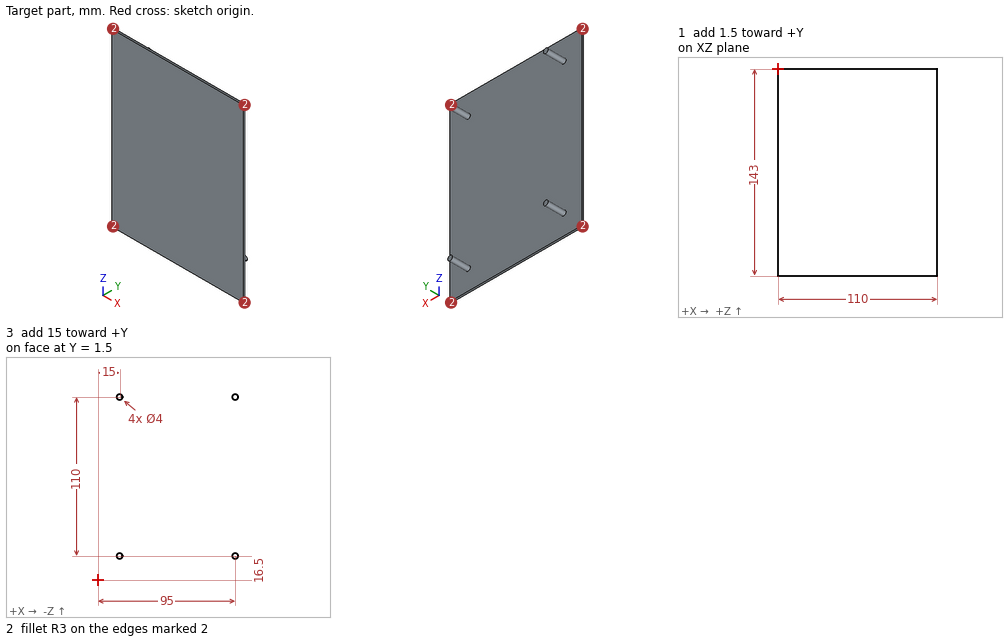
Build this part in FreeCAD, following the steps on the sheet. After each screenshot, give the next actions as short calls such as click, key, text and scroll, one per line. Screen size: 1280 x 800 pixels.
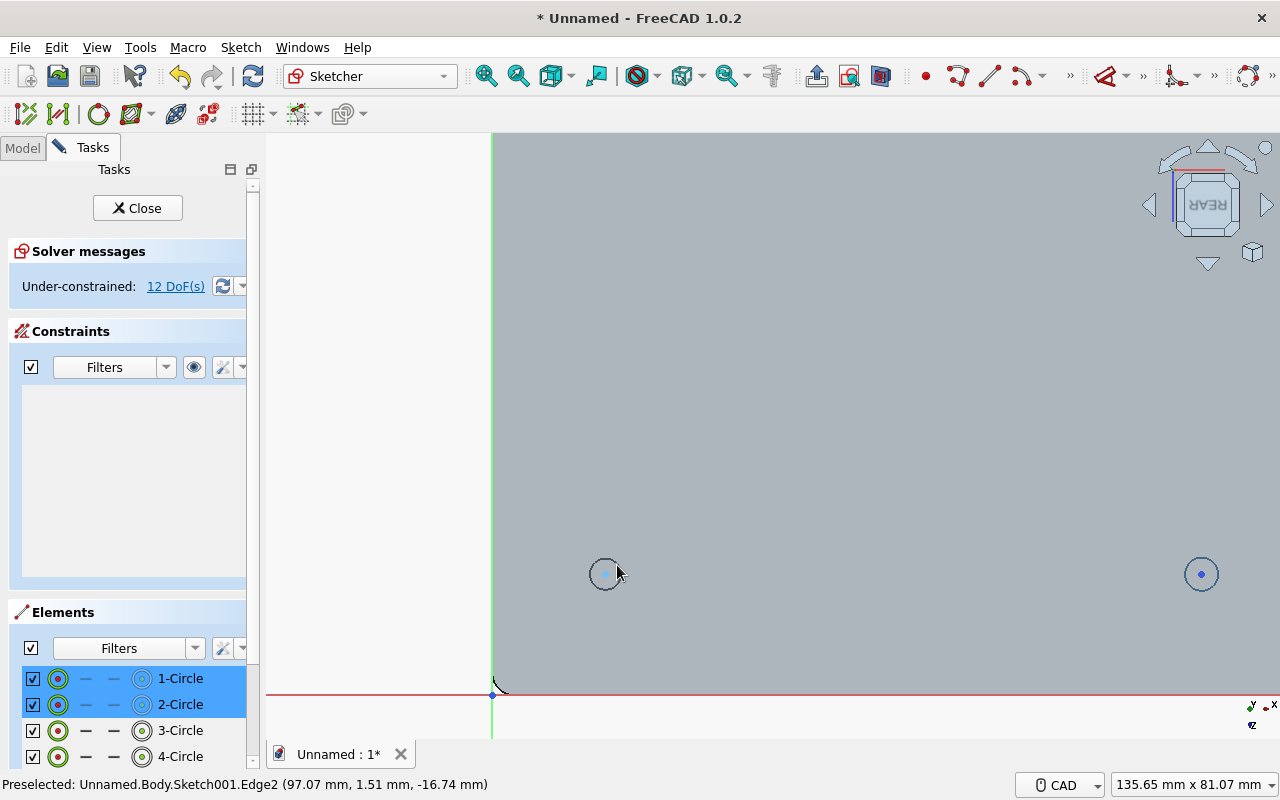
click(617, 563)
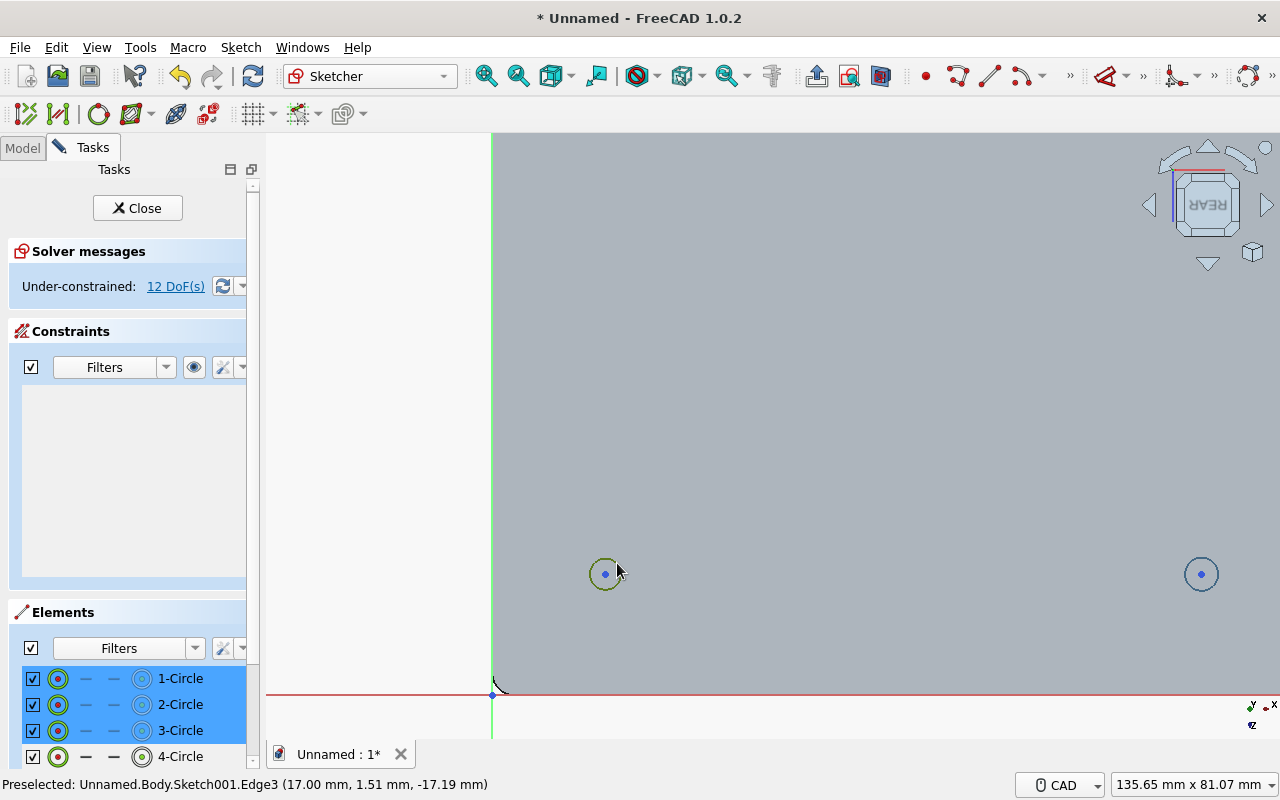
scroll(617, 565, down, 5)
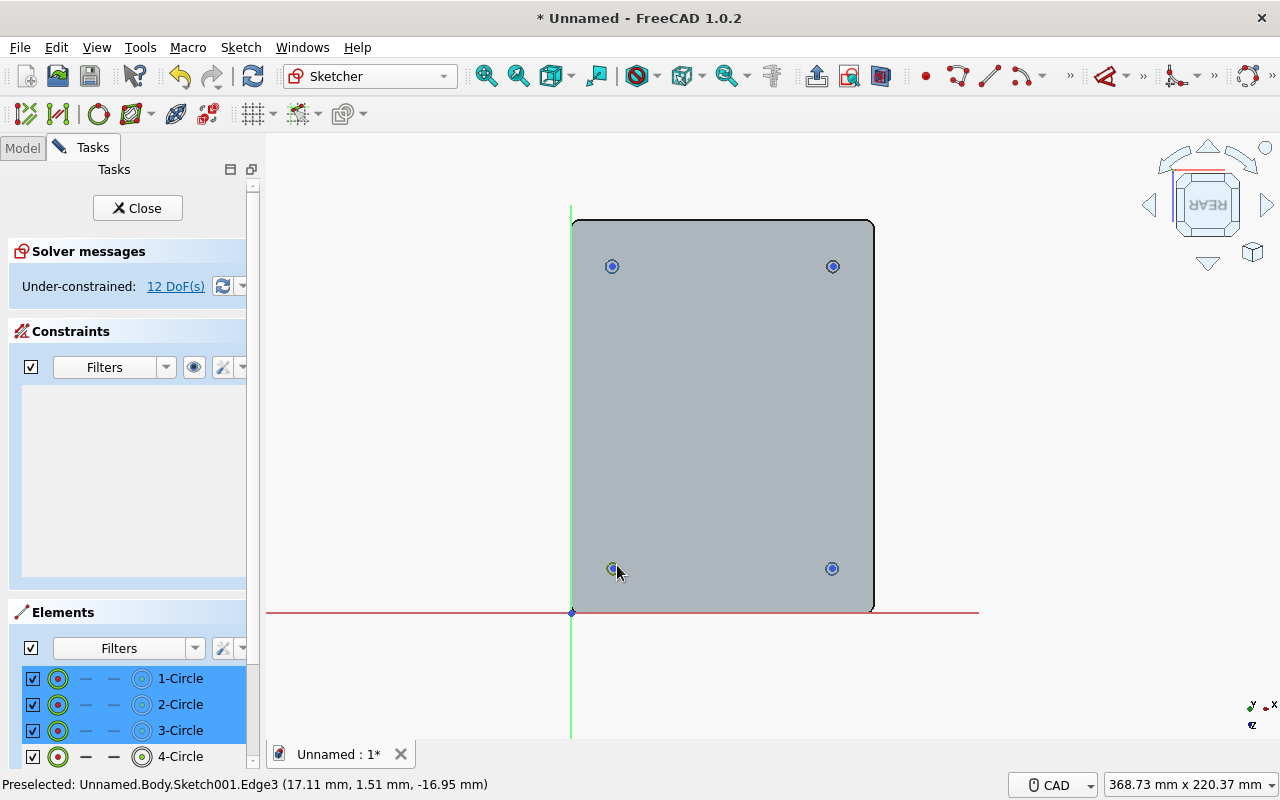
scroll(837, 262, up, 5)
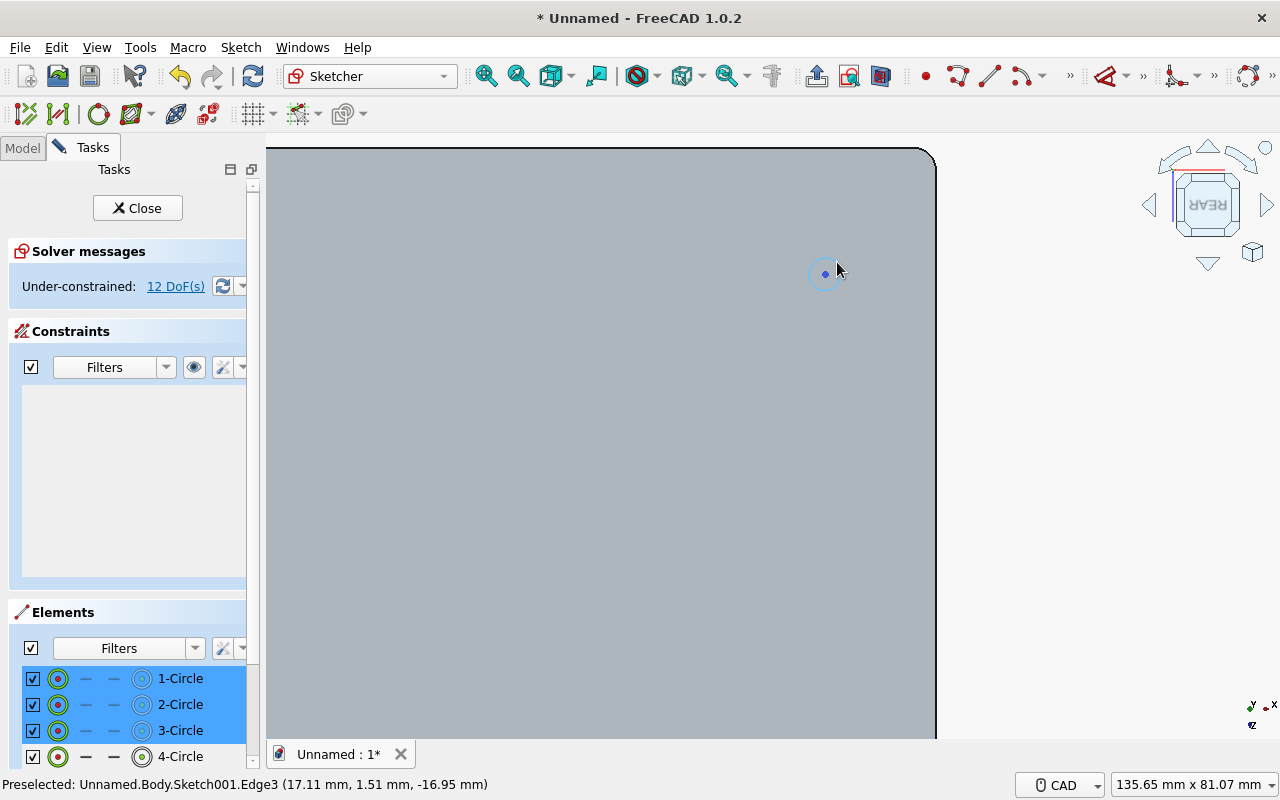
click(837, 263)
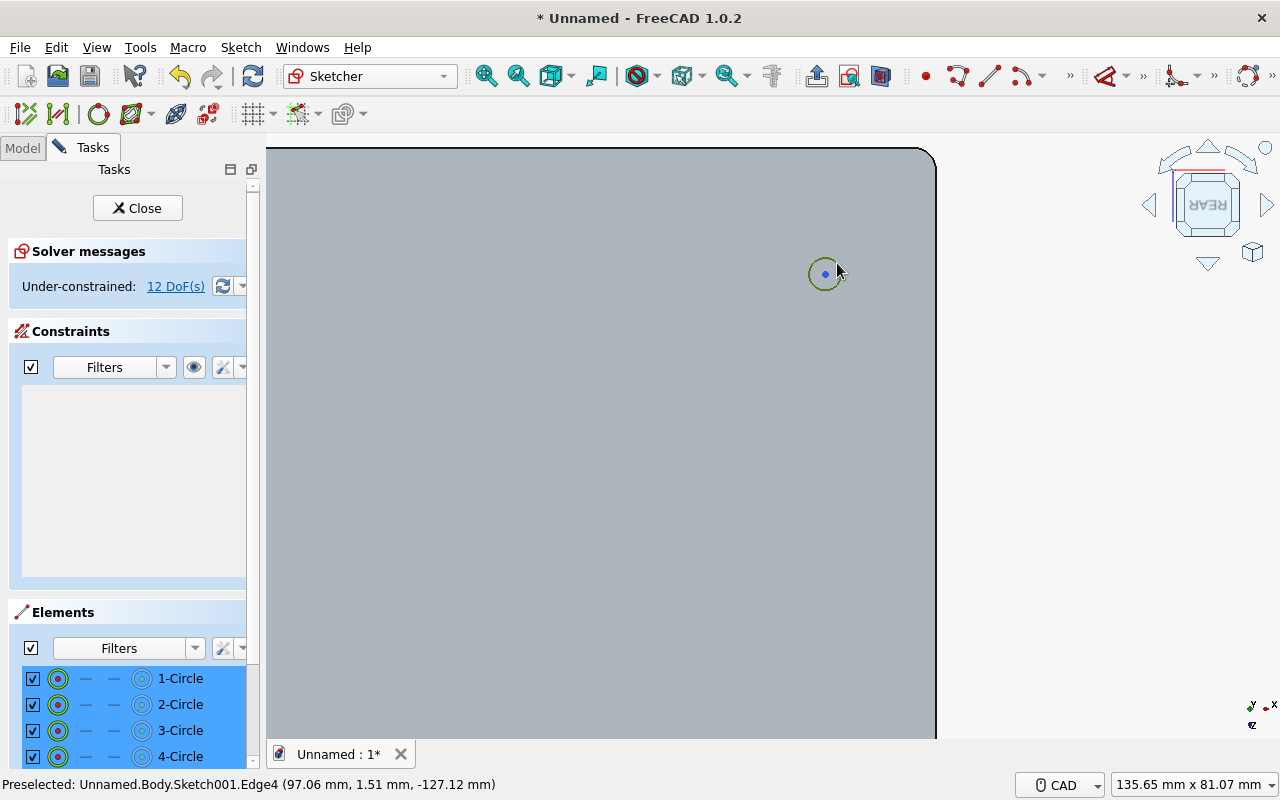
key(e)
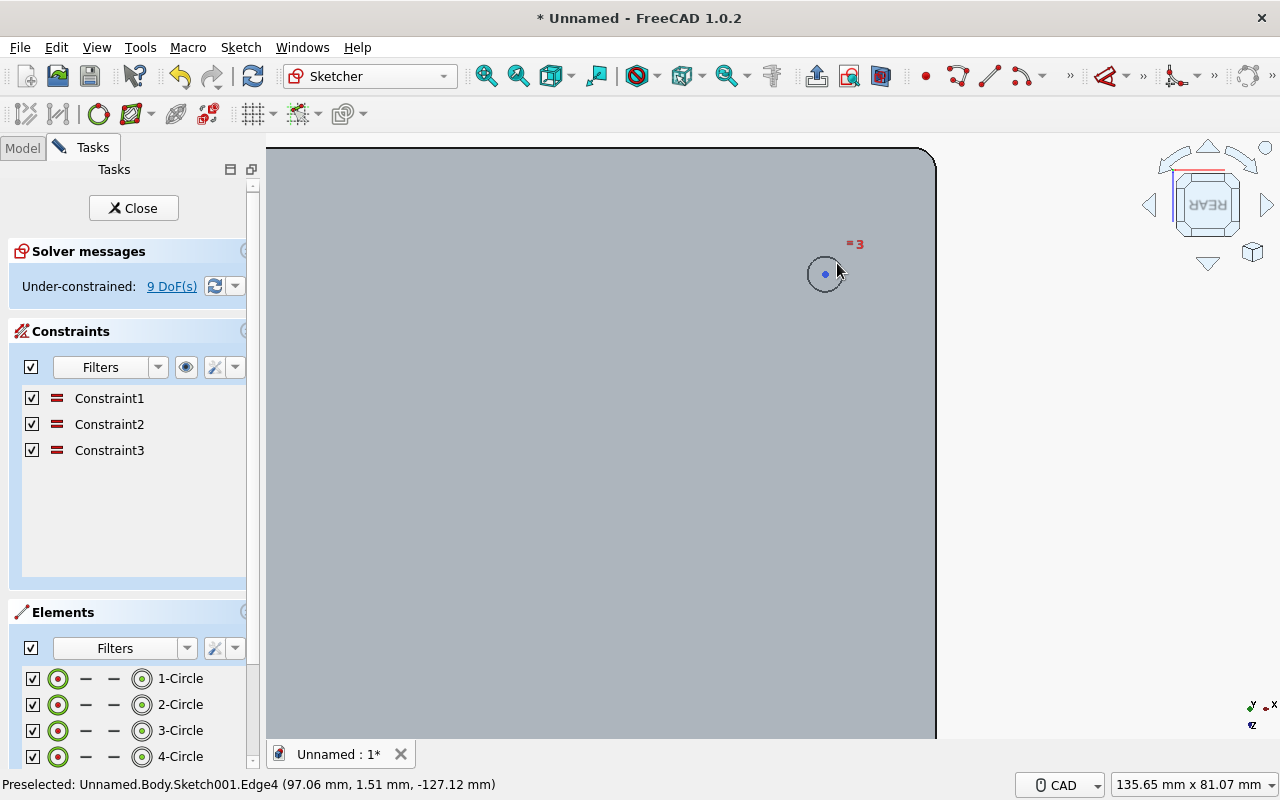
scroll(837, 261, down, 5)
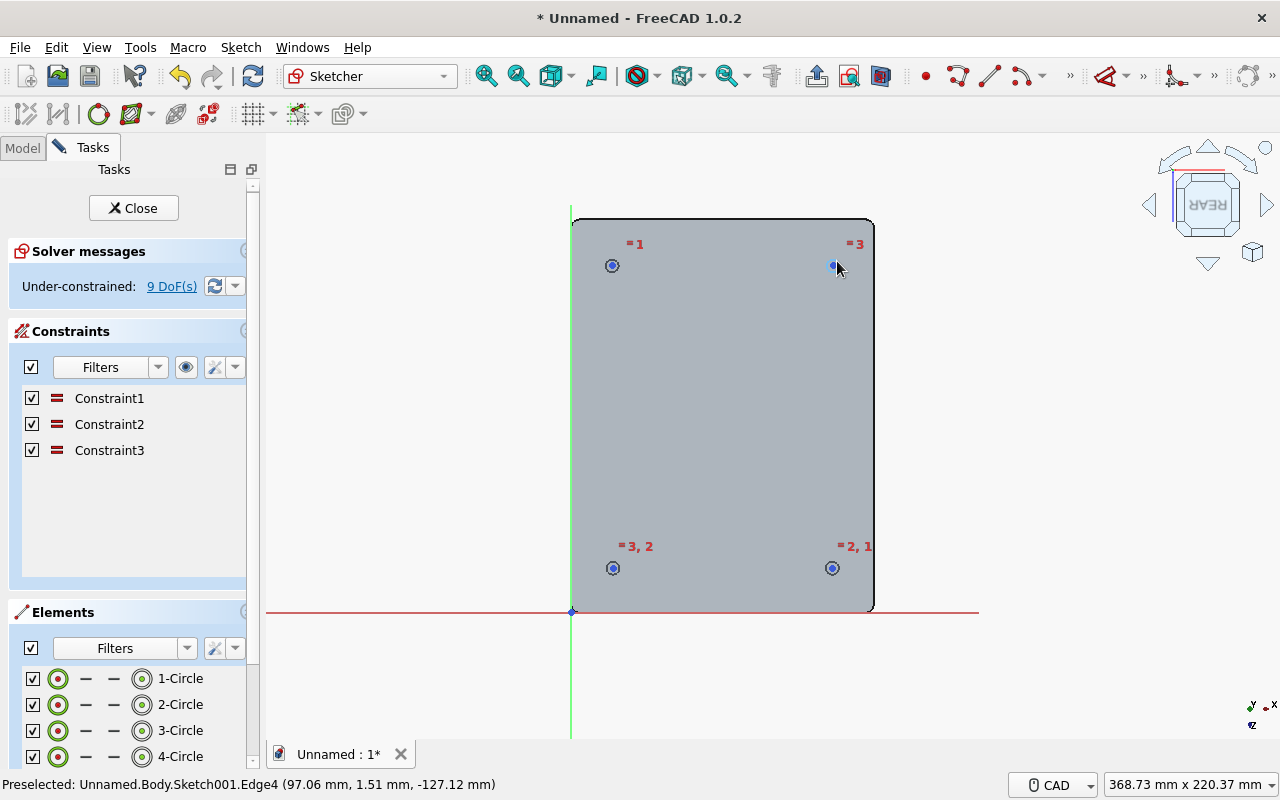
click(612, 266)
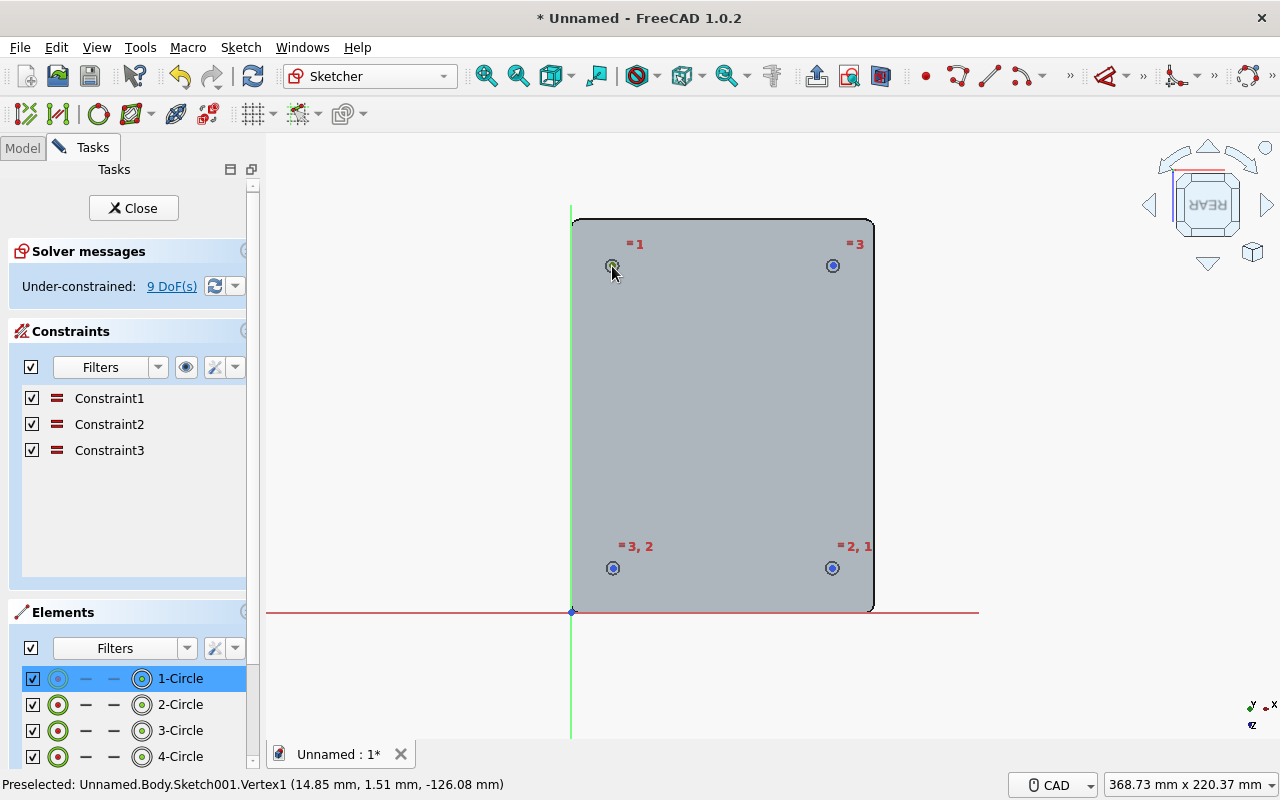
click(613, 568)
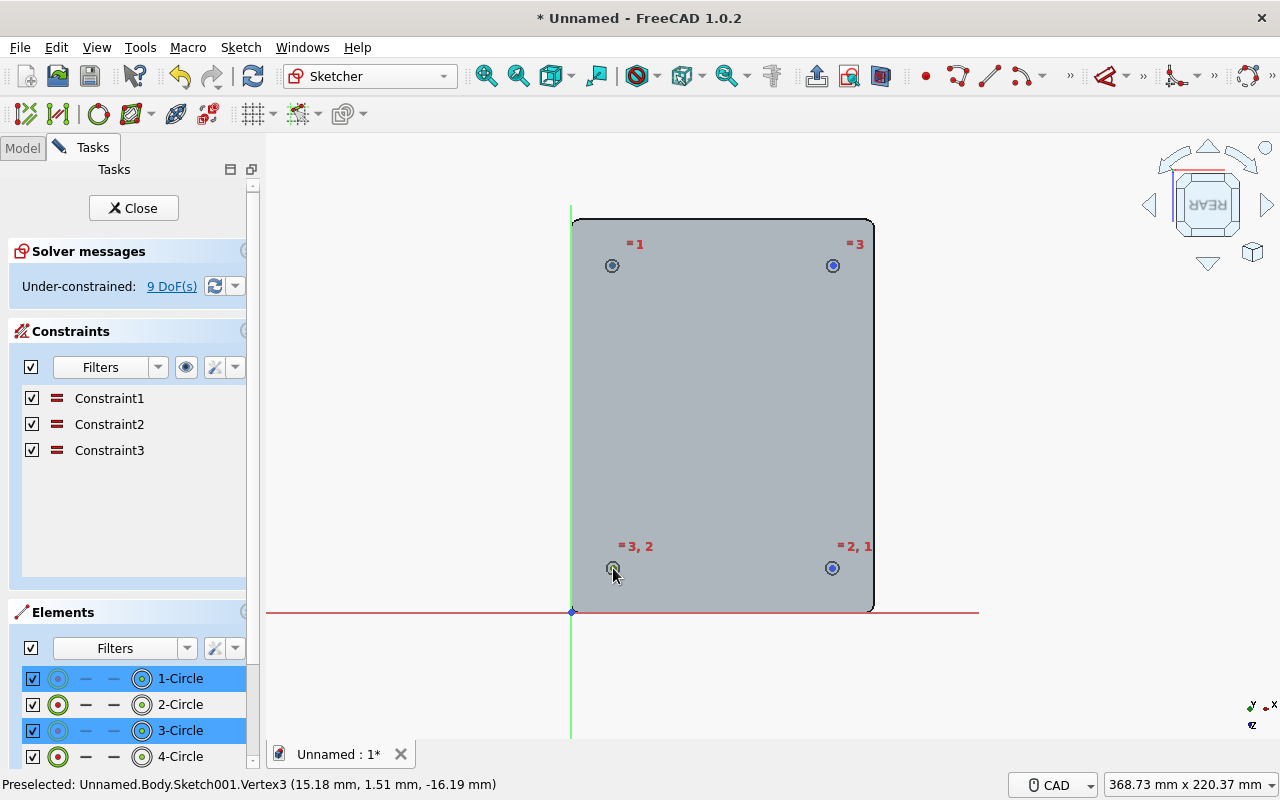
key(v)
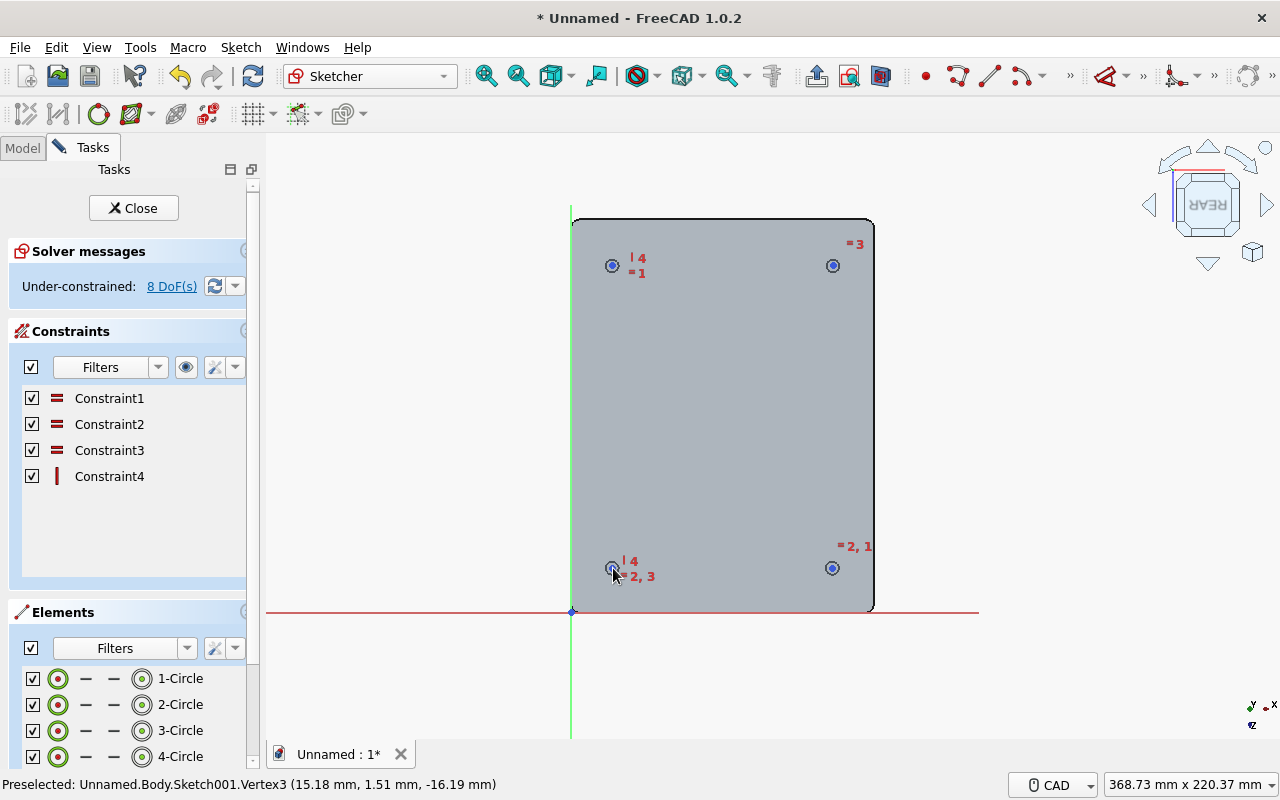
click(832, 568)